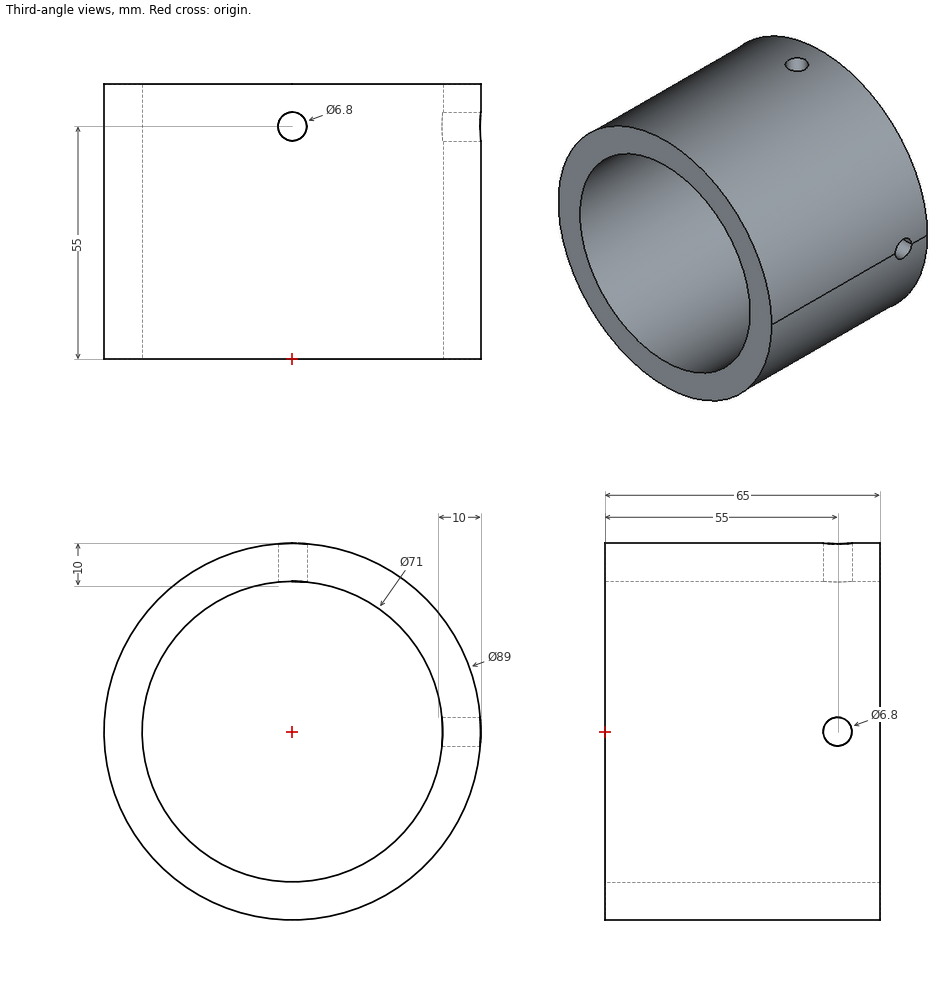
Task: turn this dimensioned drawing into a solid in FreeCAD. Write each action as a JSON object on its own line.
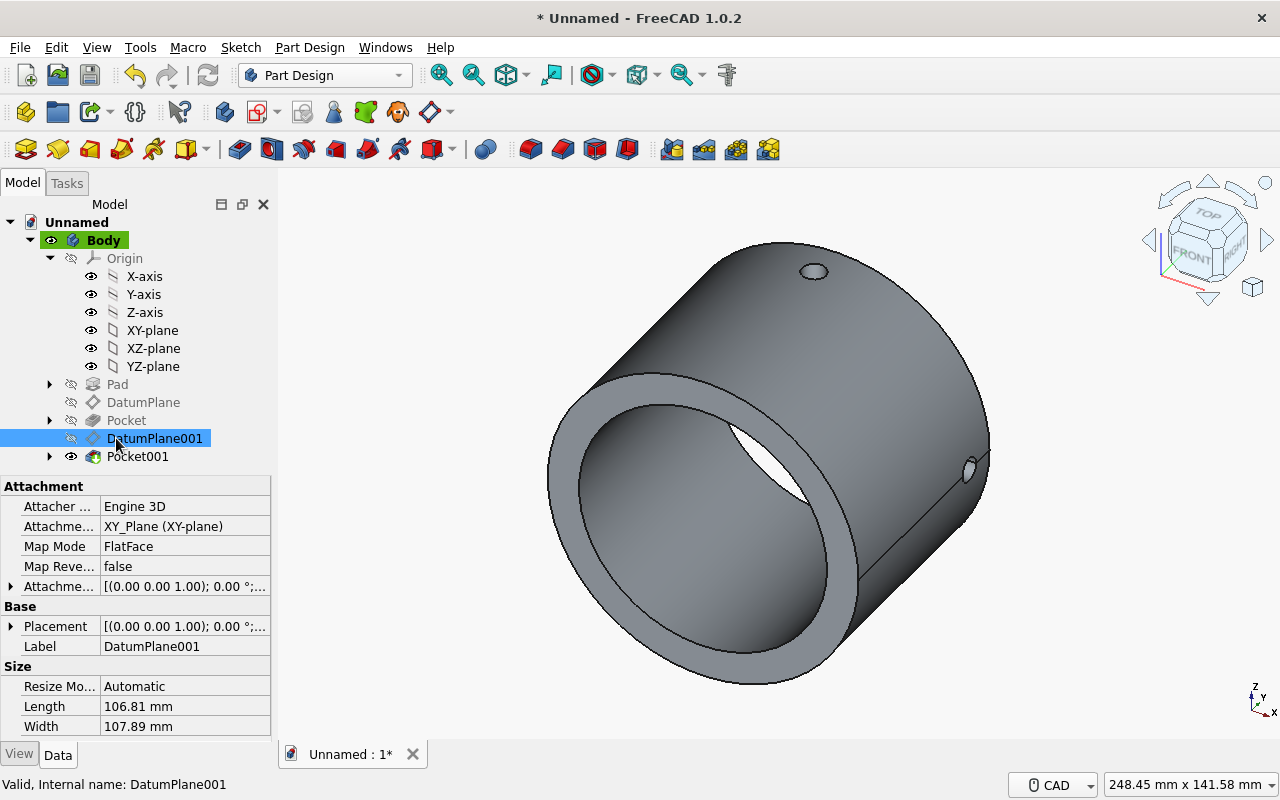
{"action": "key", "text": "0"}